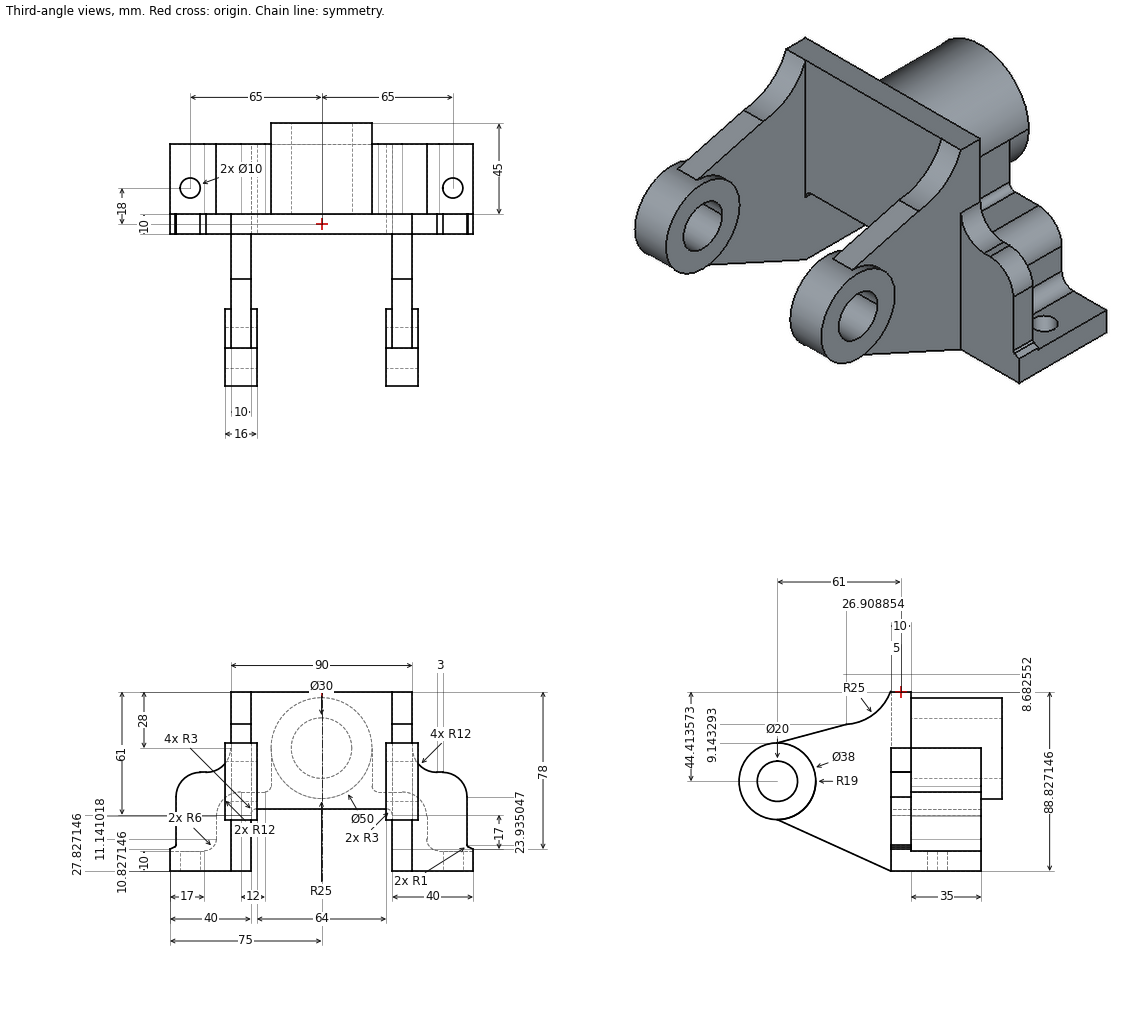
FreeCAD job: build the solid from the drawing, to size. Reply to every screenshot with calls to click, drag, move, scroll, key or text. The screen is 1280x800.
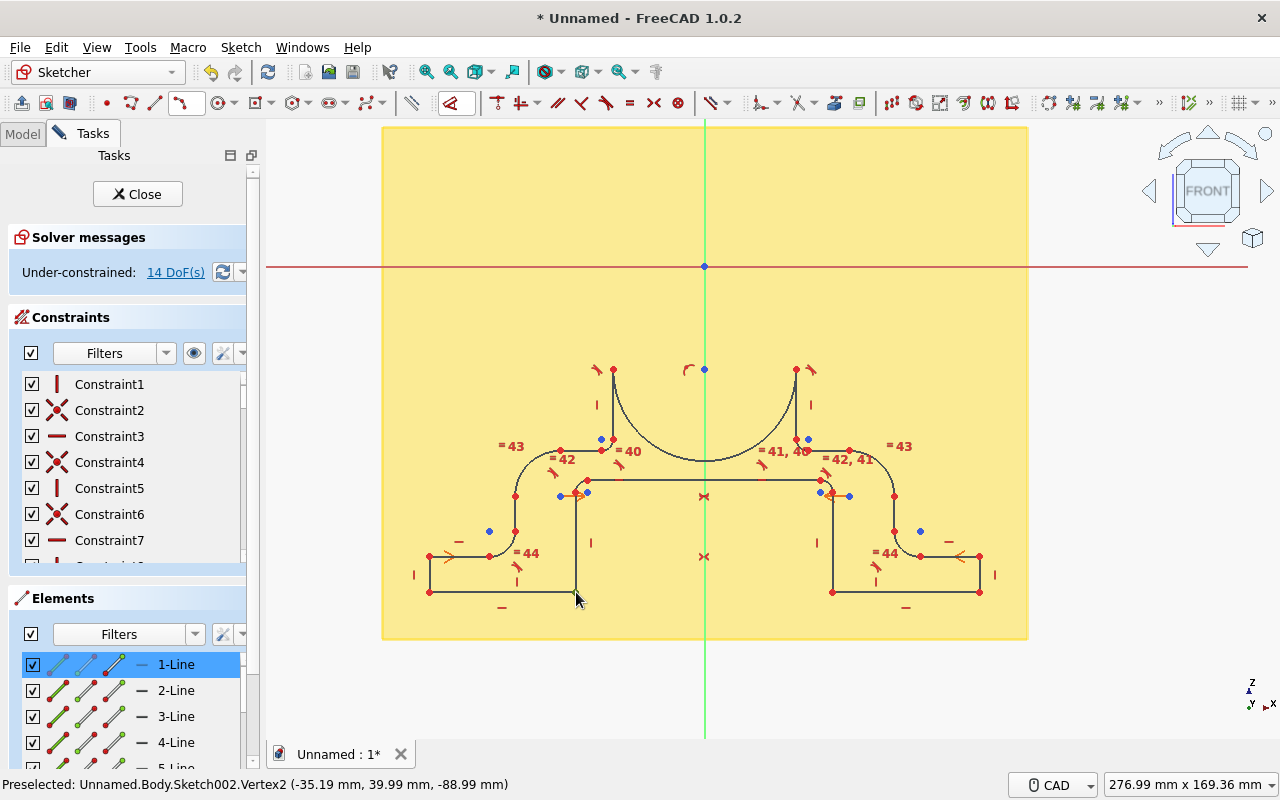
click(833, 592)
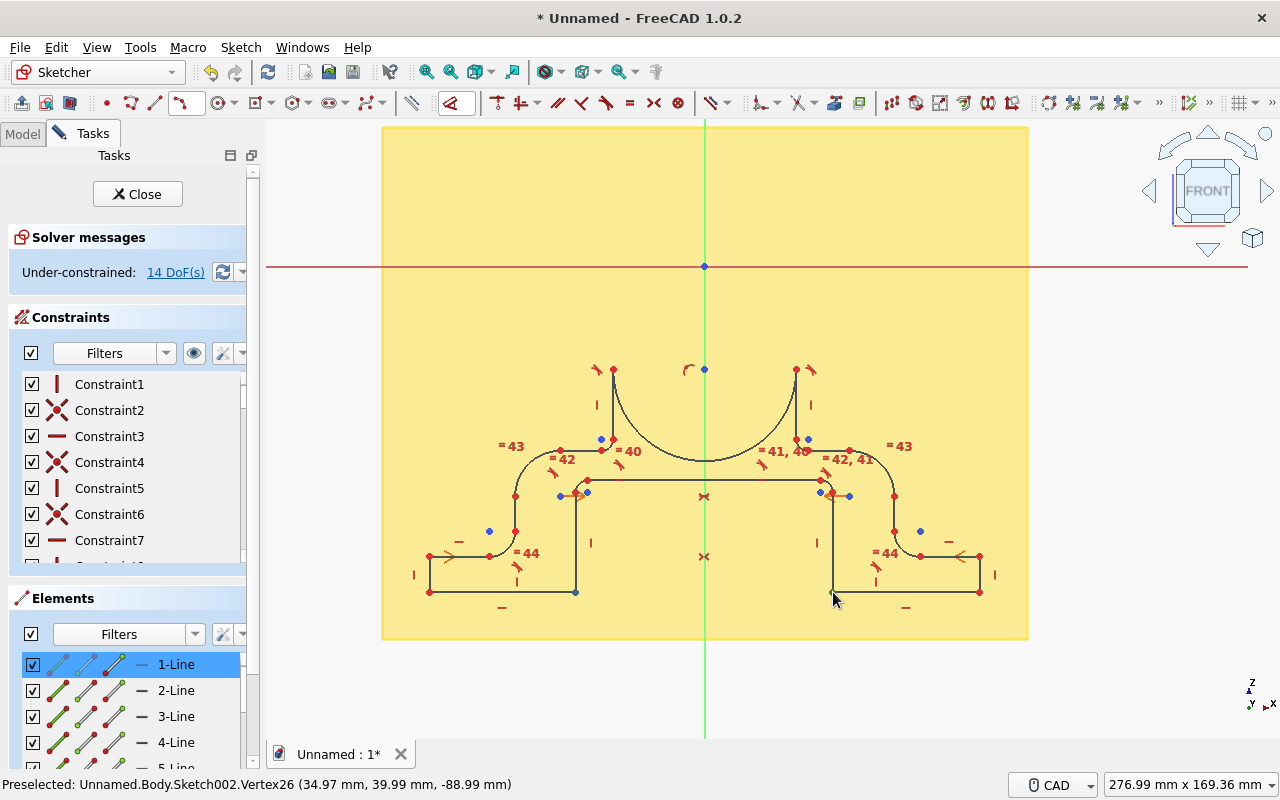
click(705, 671)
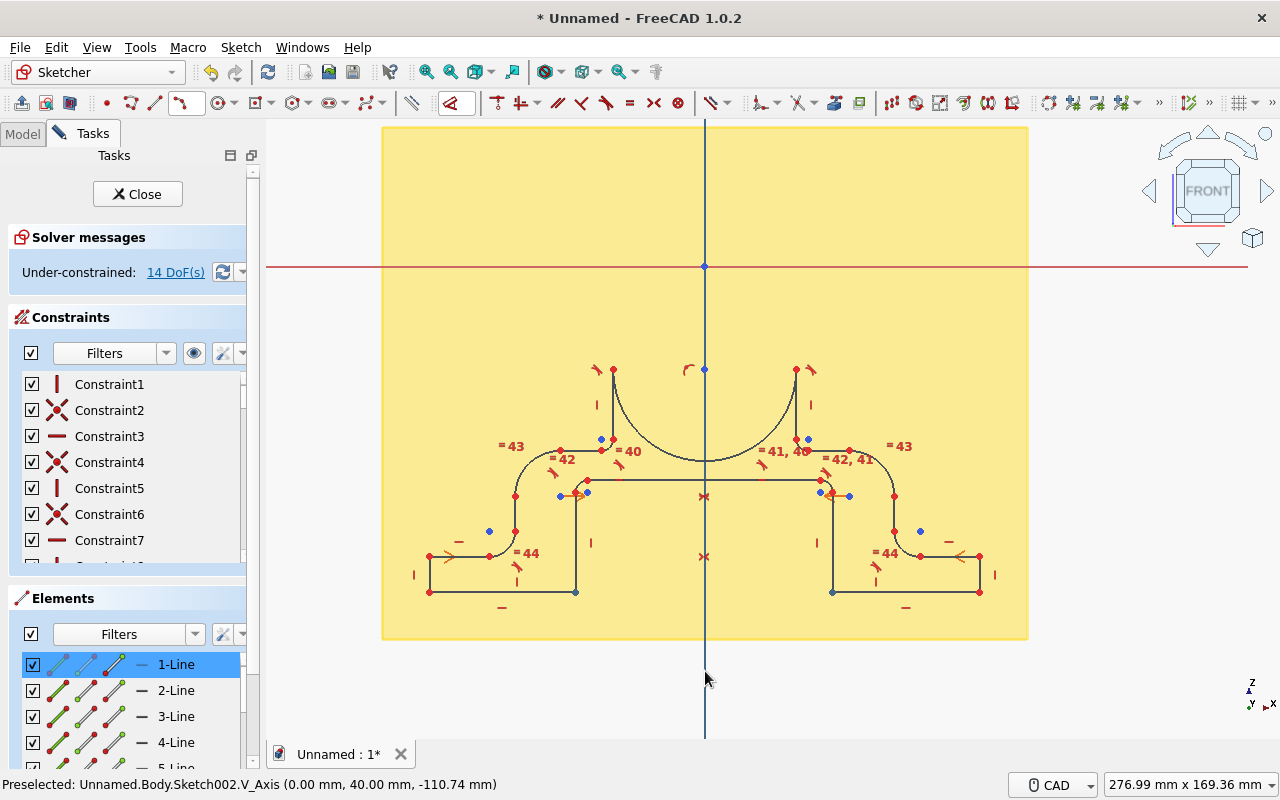
key(s)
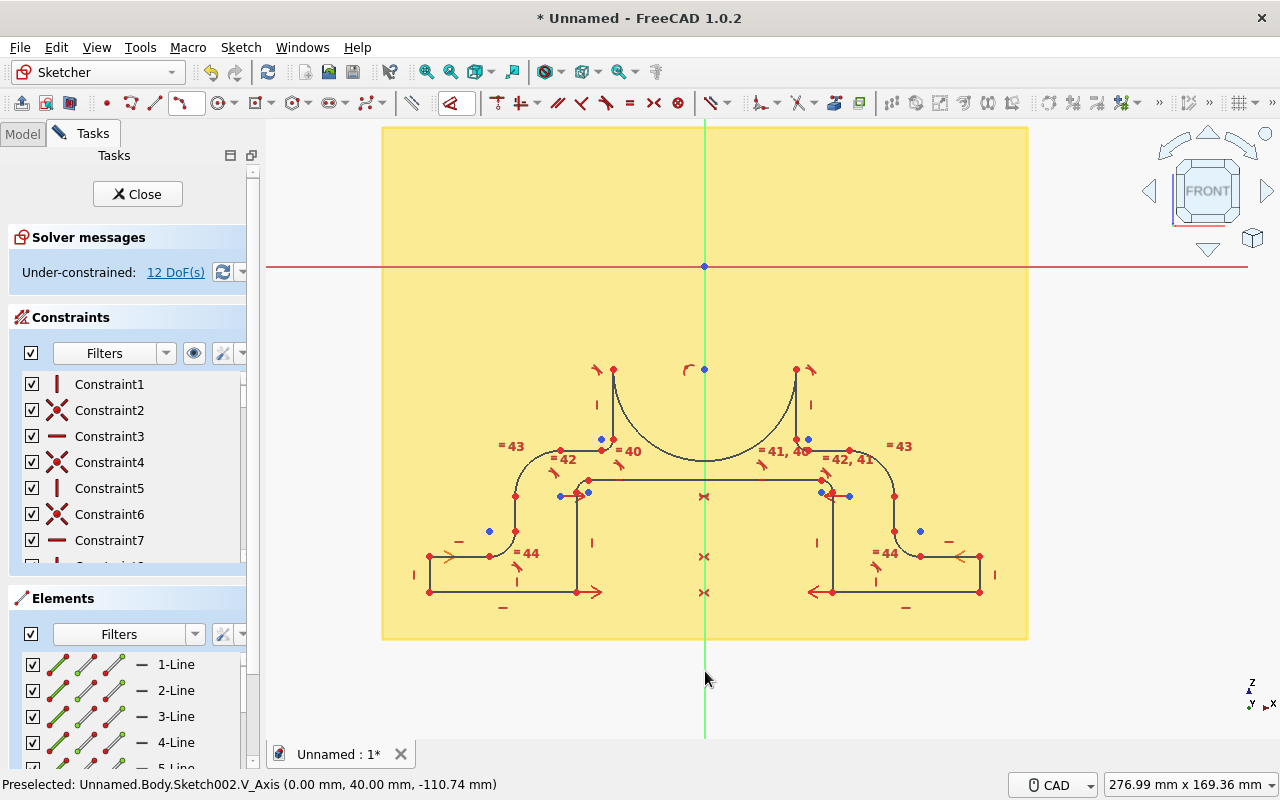
click(450, 104)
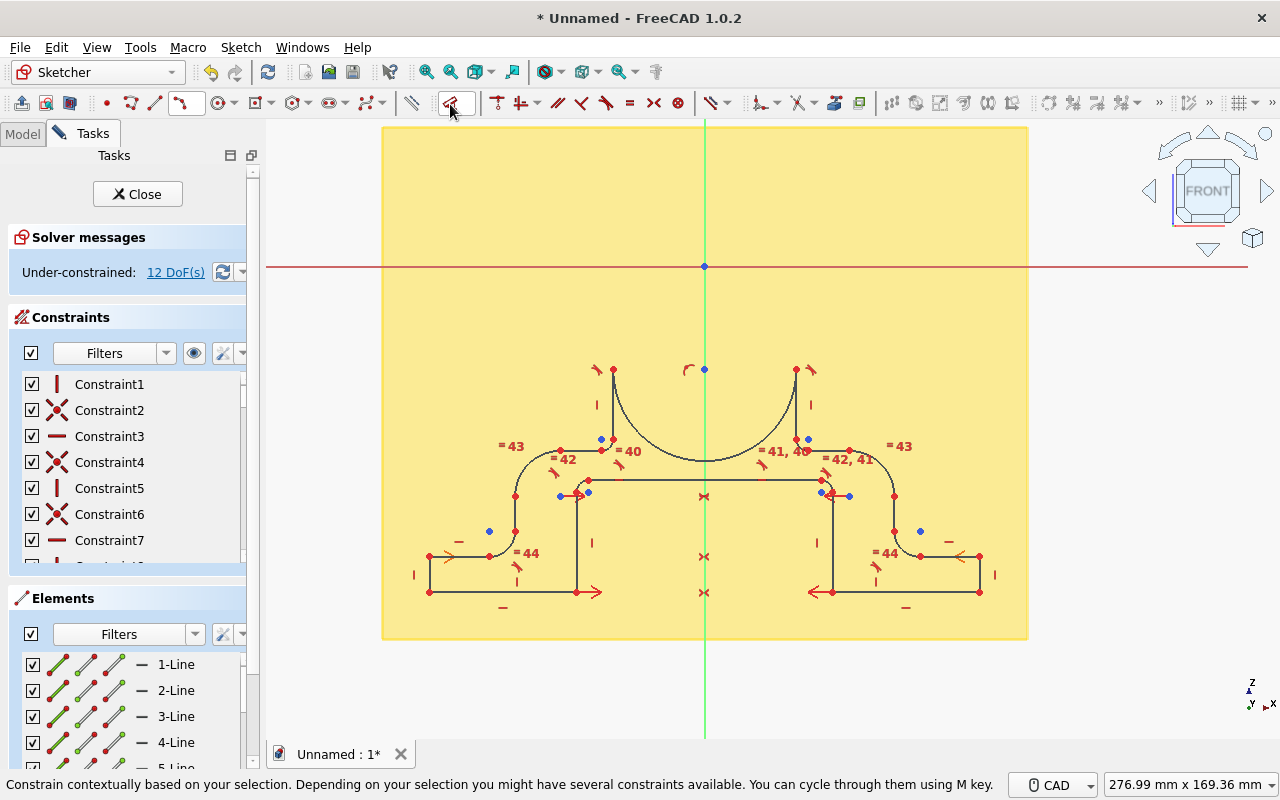
scroll(501, 554, up, 3)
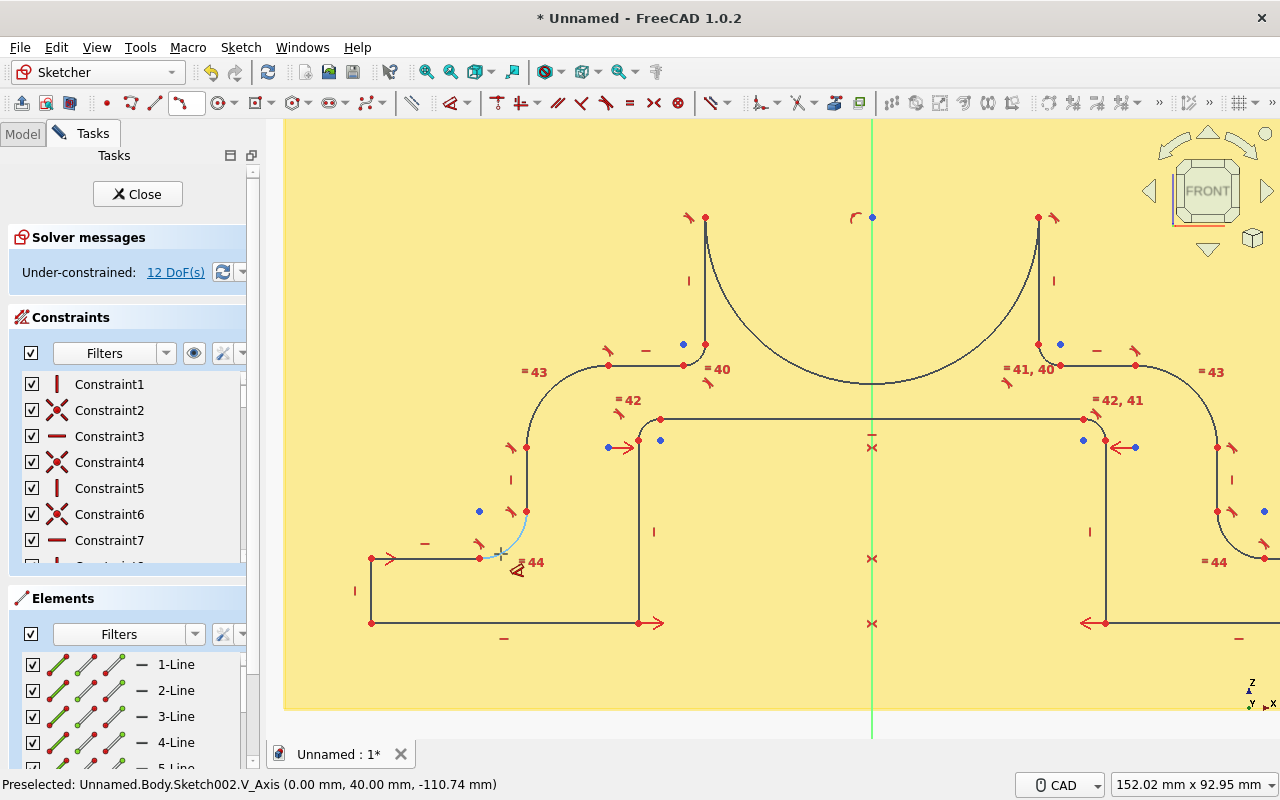
click(501, 554)
click(515, 583)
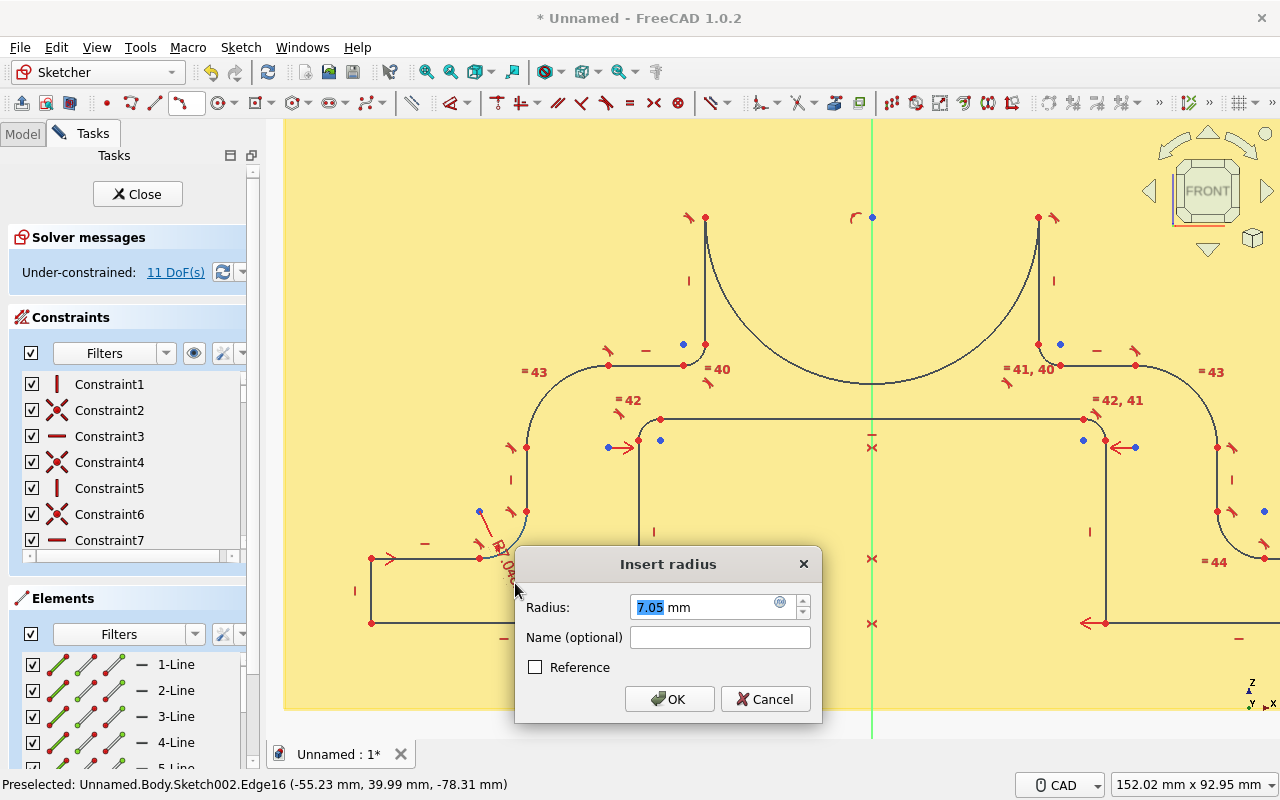
text(6)
key(Return)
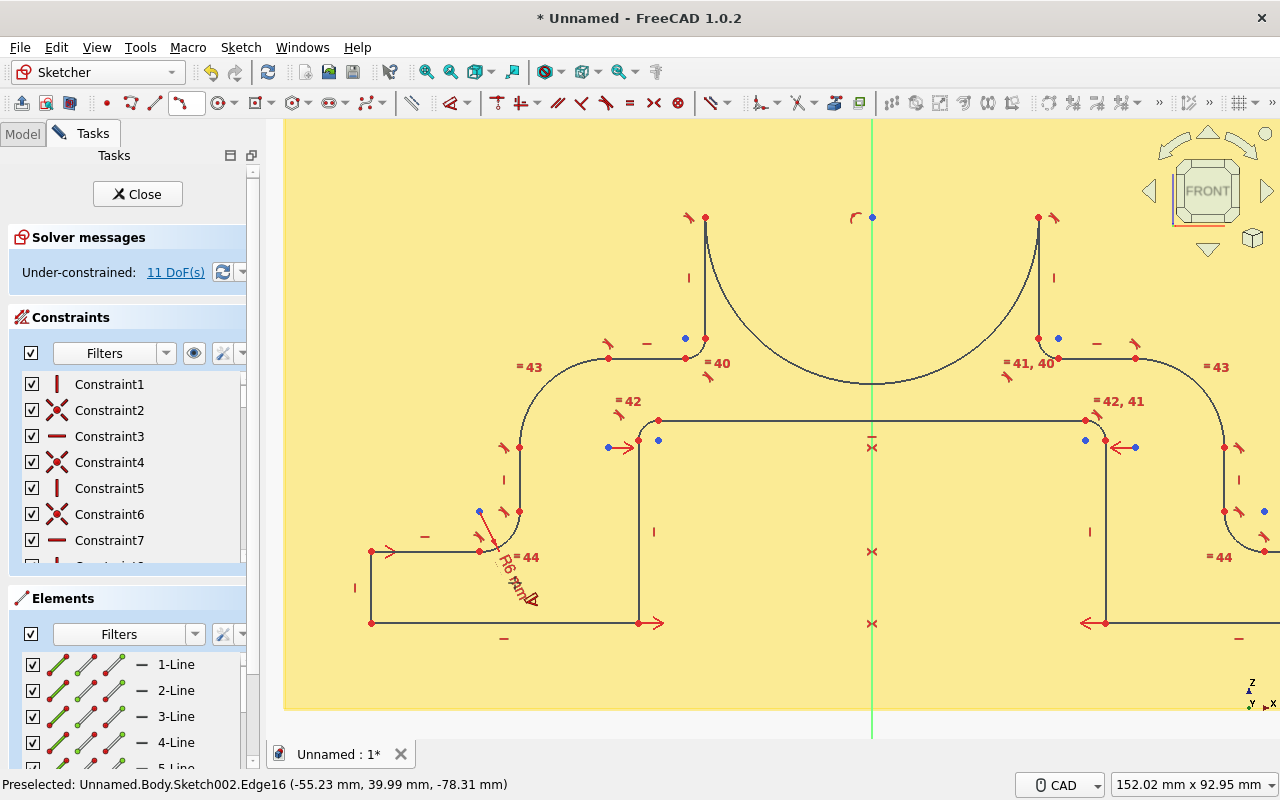
click(568, 368)
click(553, 340)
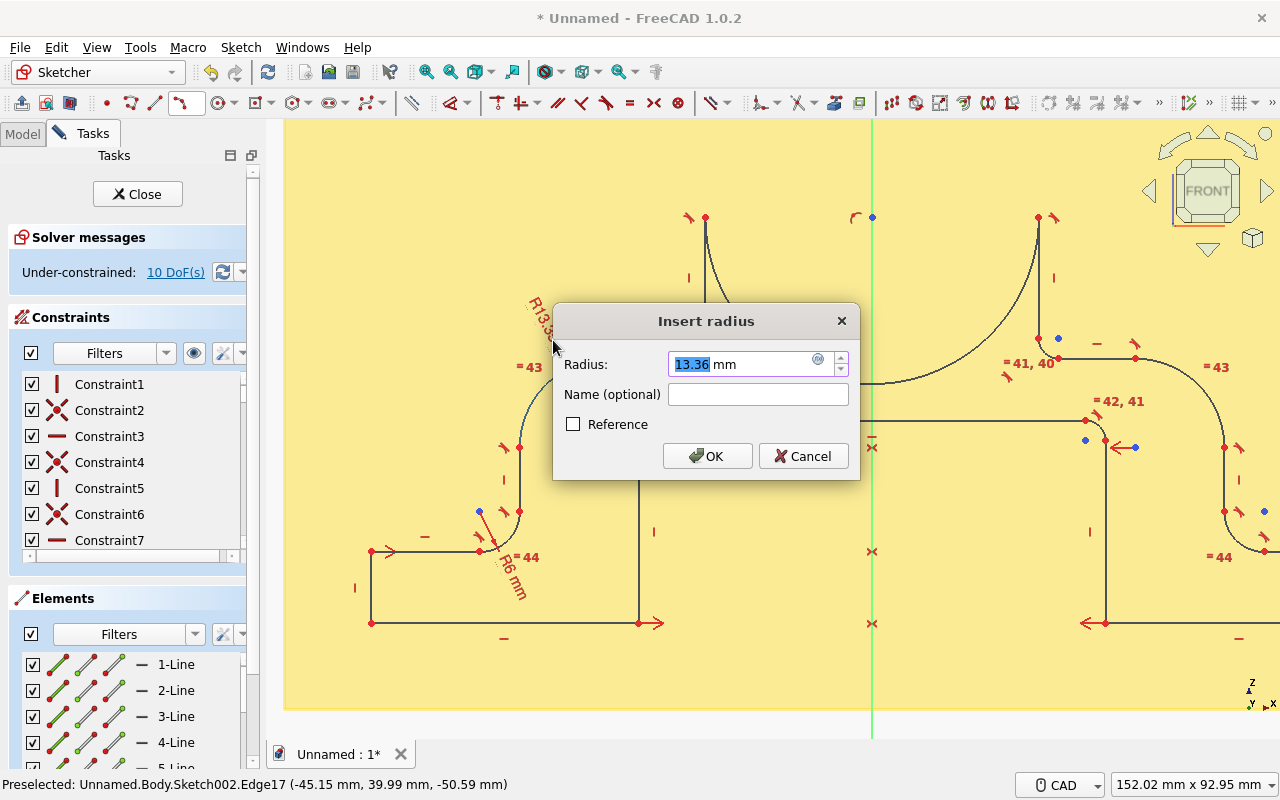
text(12)
key(Return)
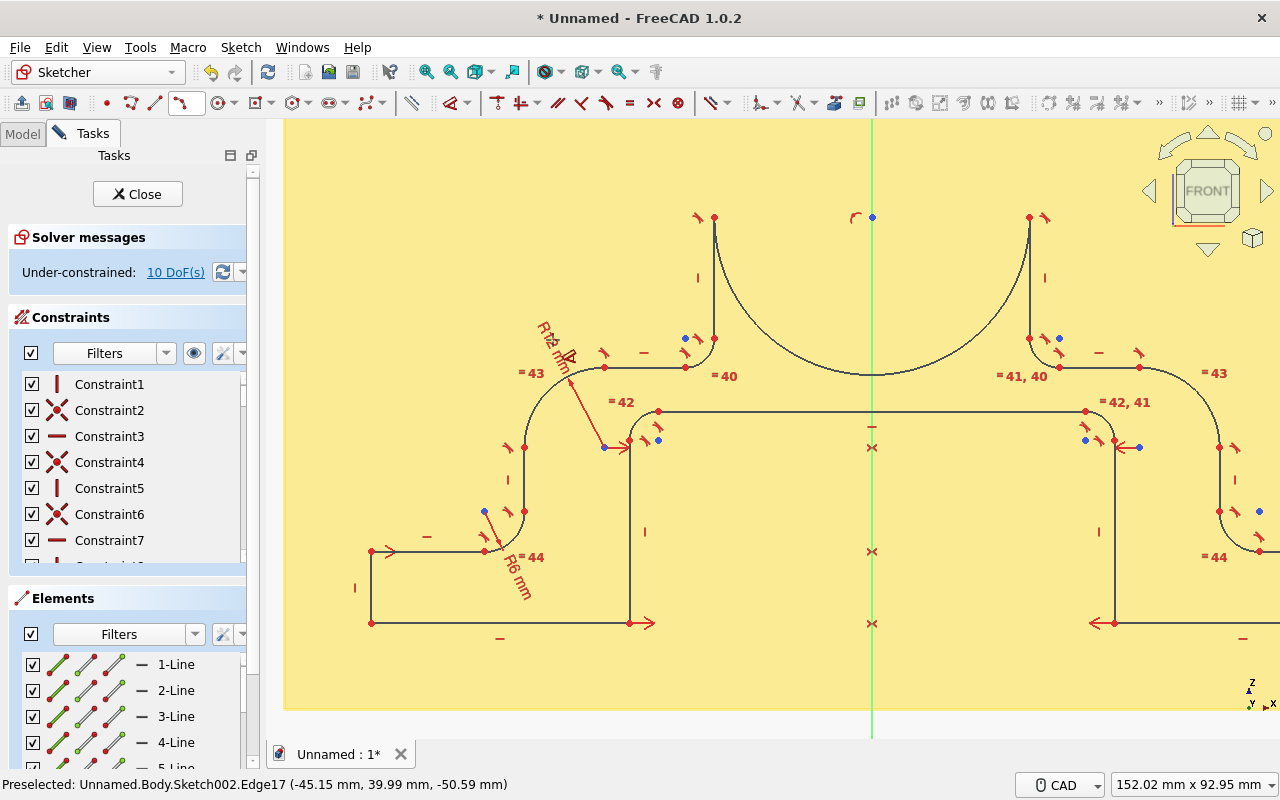
scroll(698, 365, up, 4)